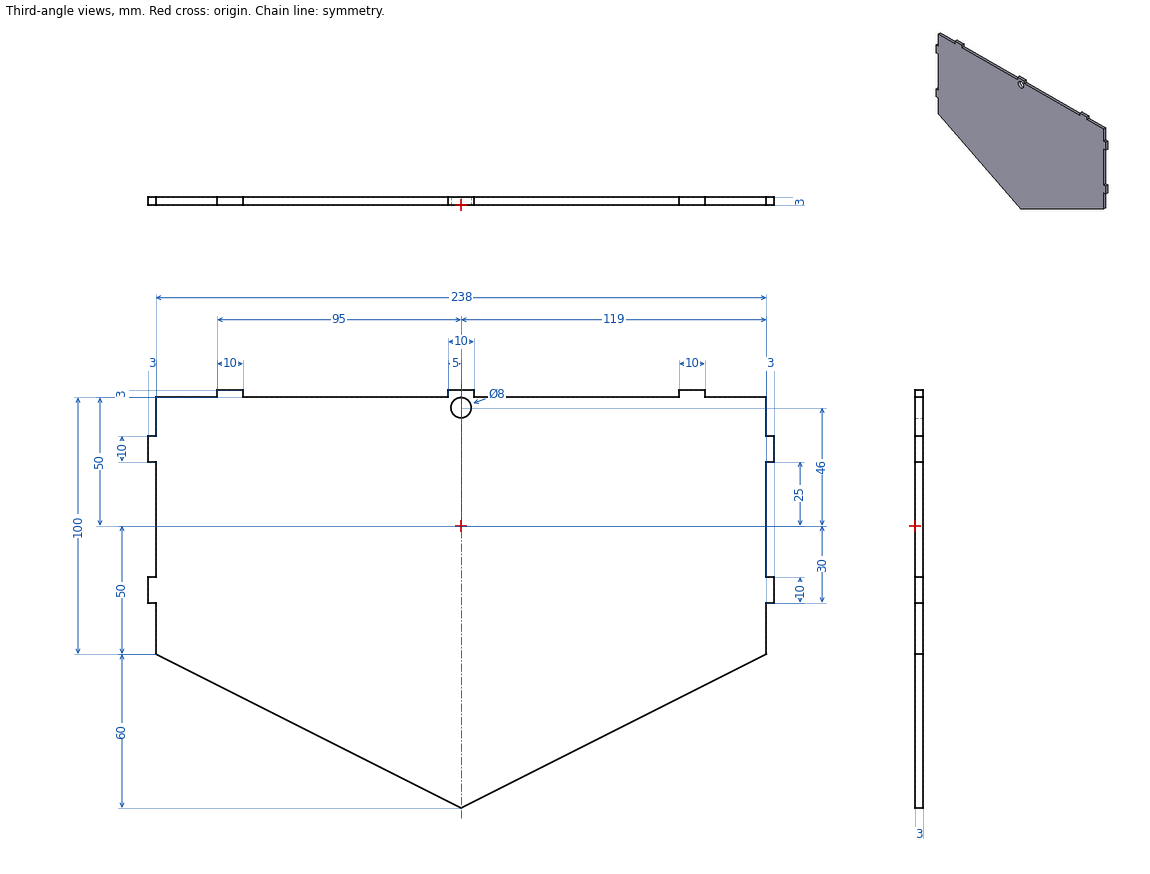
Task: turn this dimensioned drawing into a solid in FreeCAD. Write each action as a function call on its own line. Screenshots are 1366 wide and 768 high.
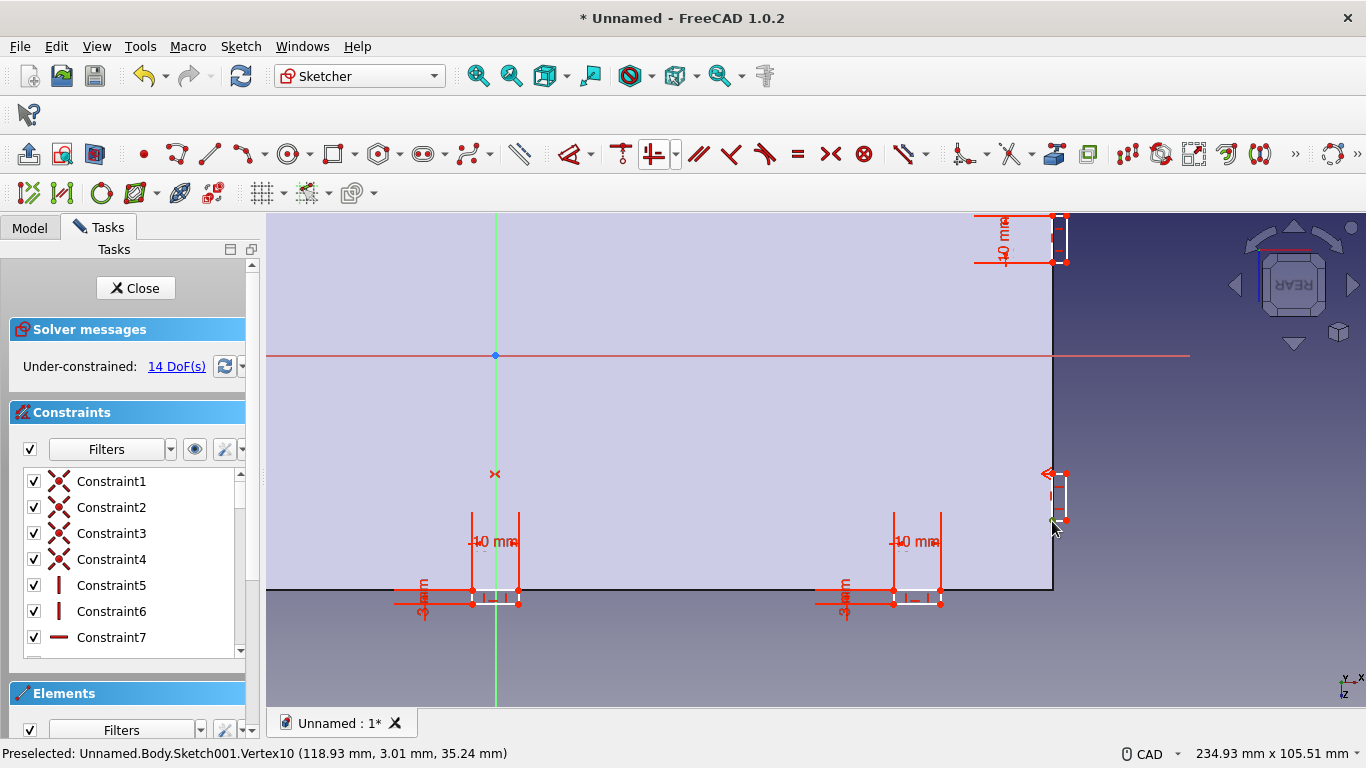
scroll(1054, 521, down, 3)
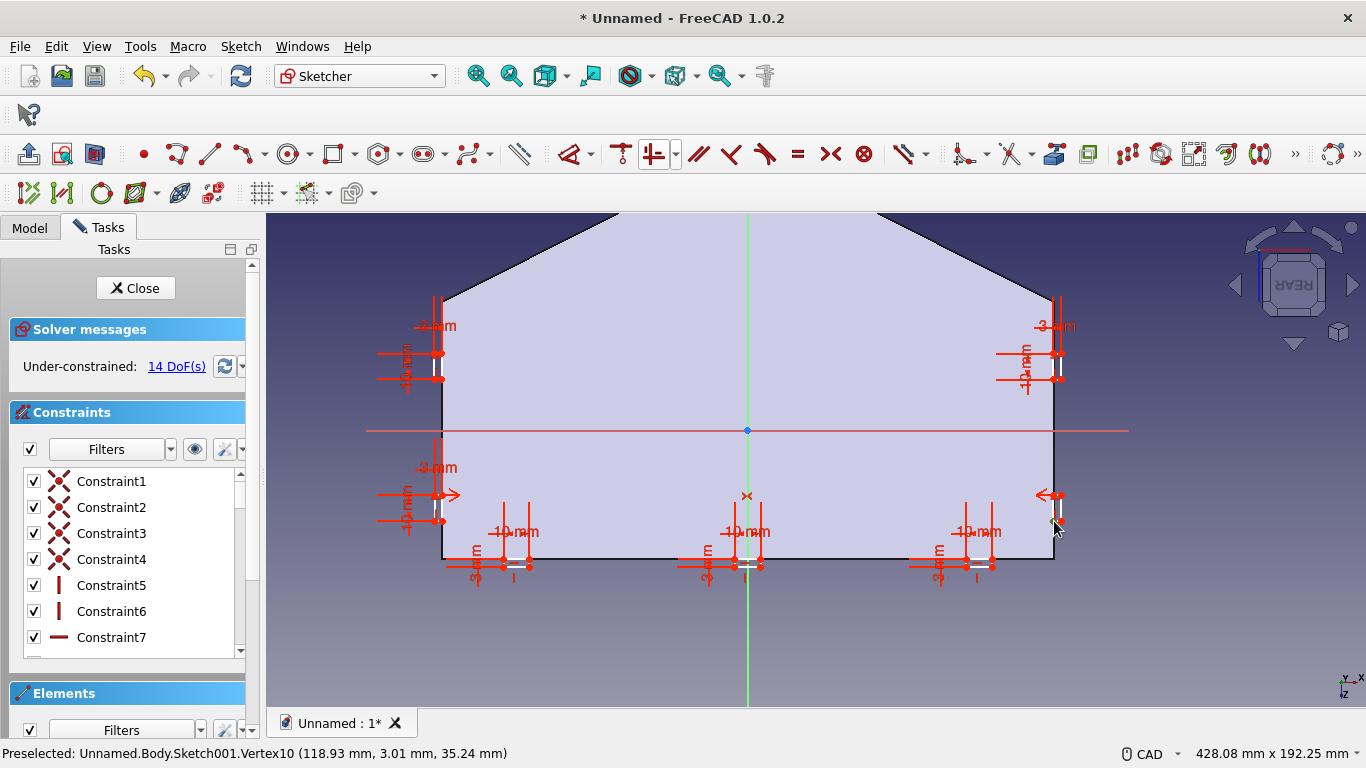
scroll(442, 521, up, 3)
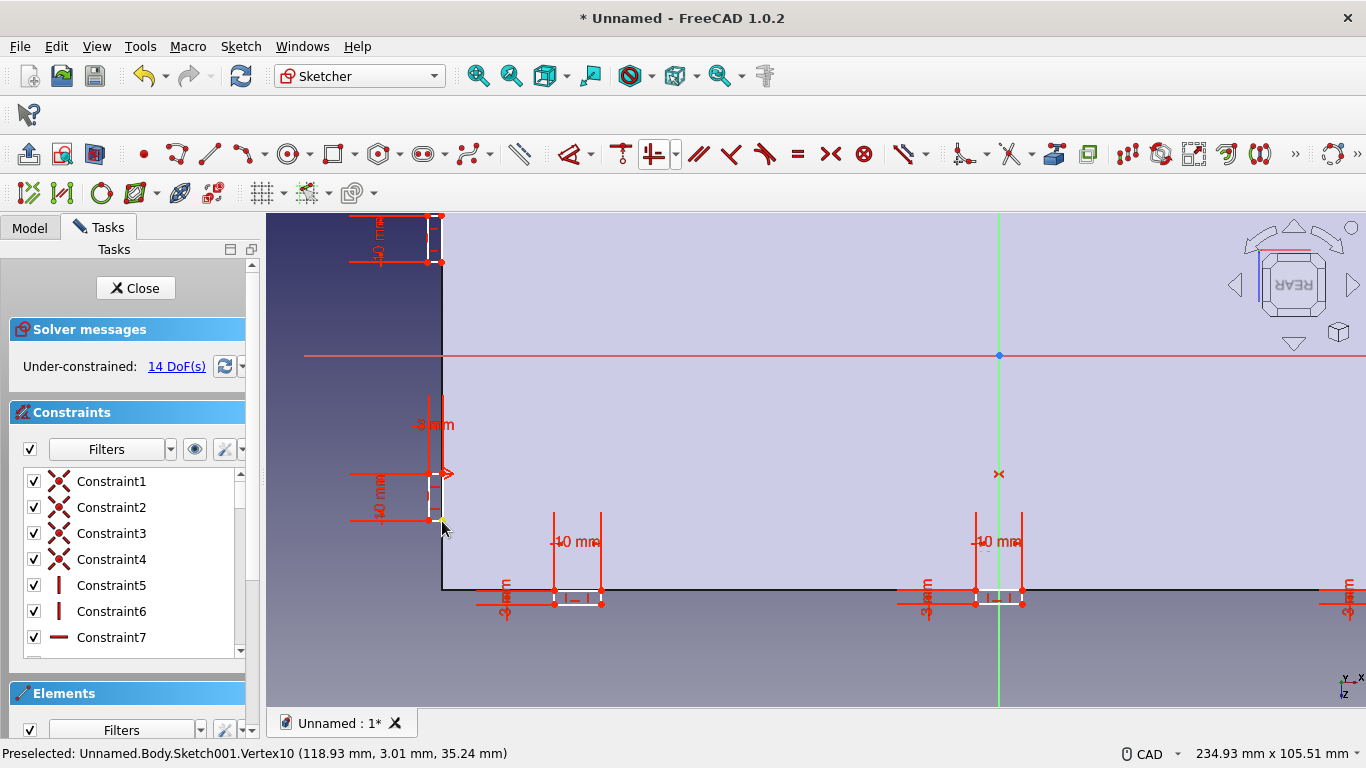
click(443, 521)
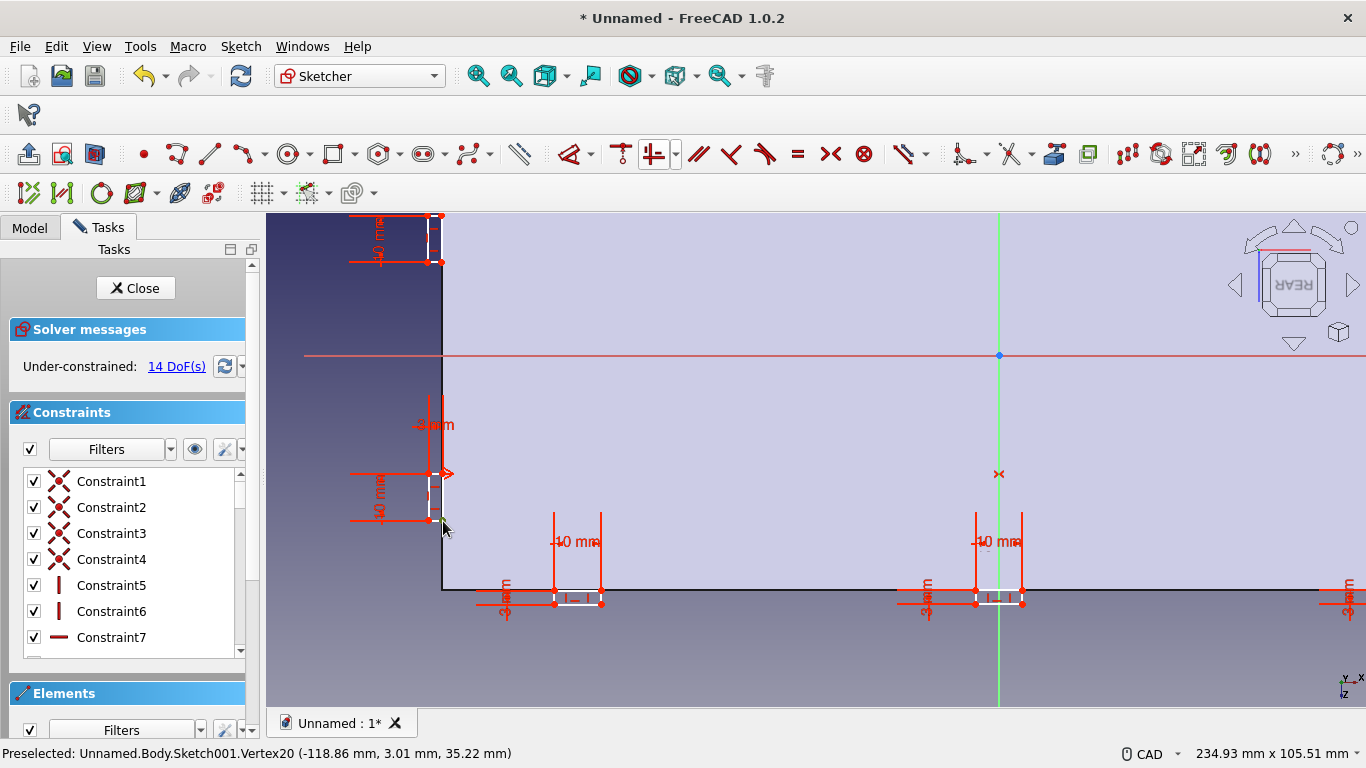
click(999, 648)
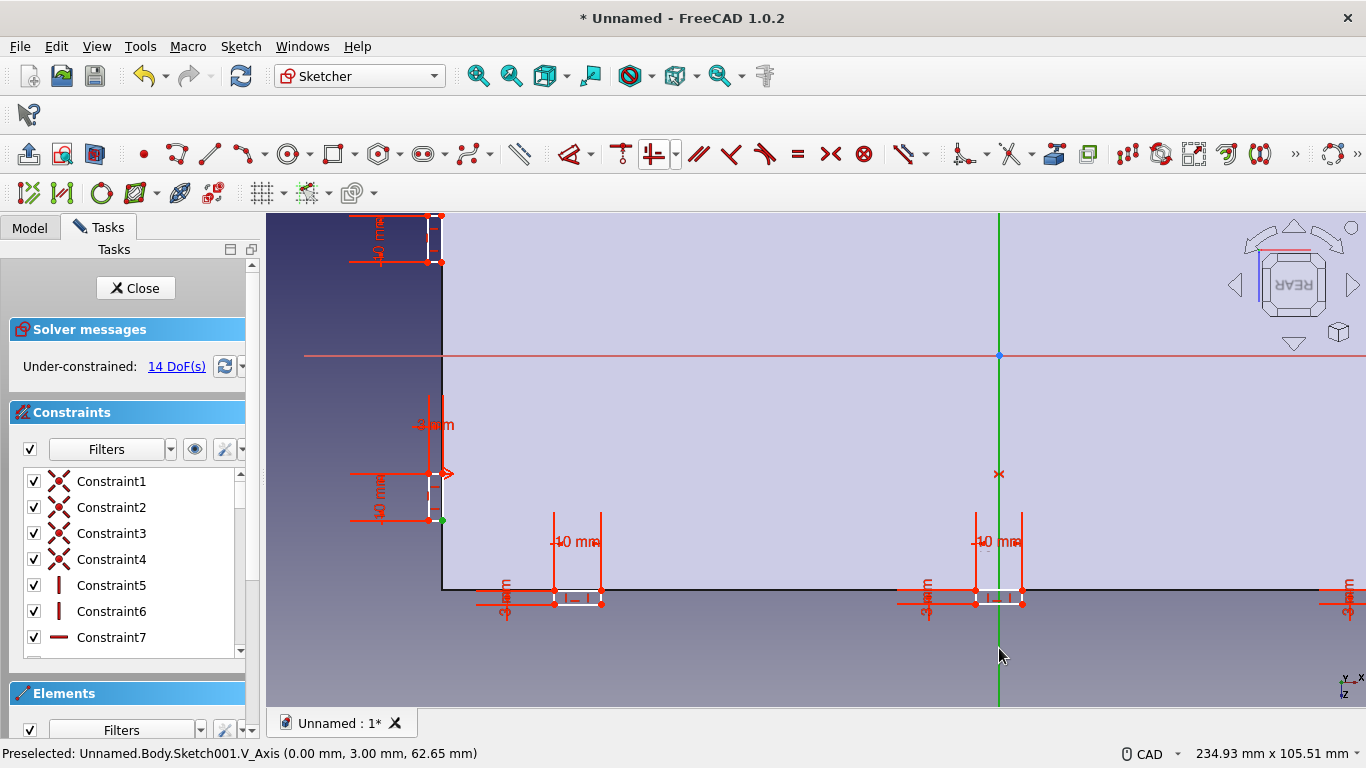
click(831, 154)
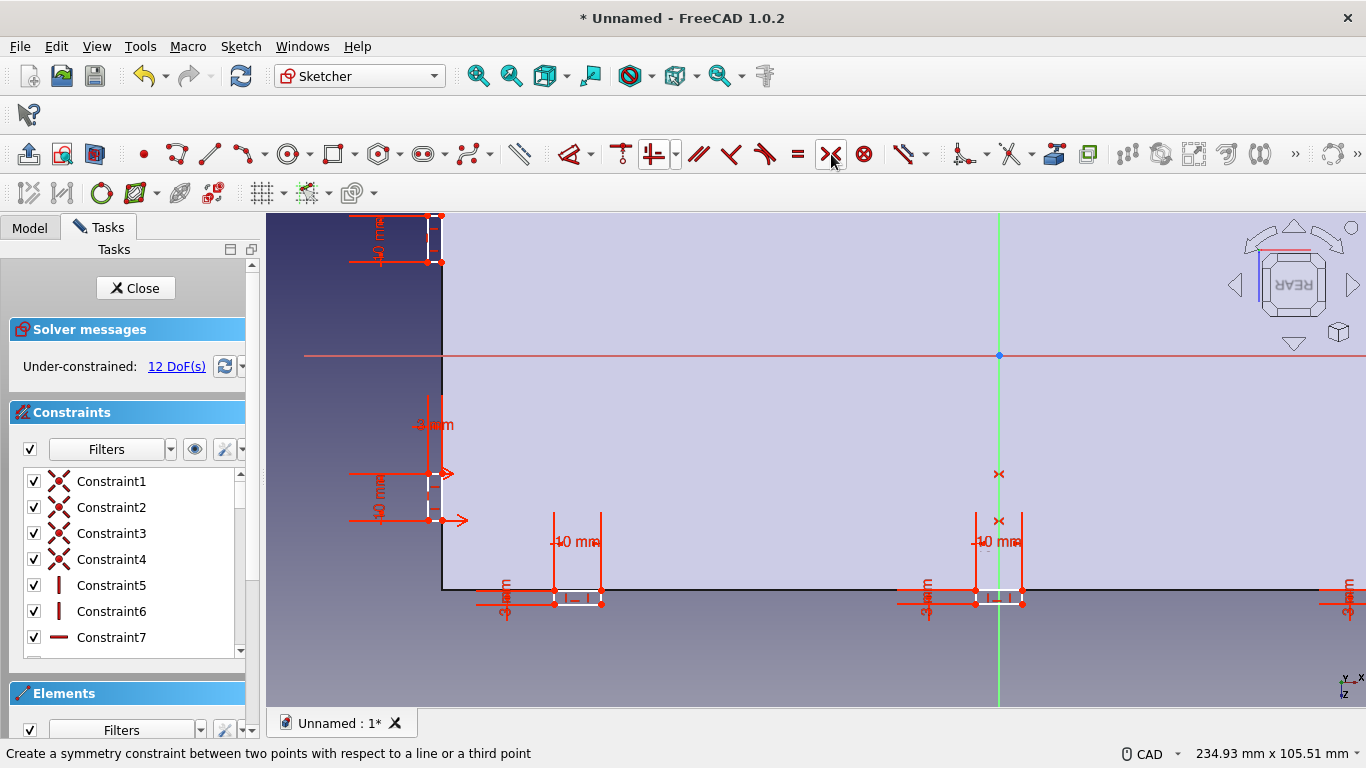
scroll(441, 521, down, 3)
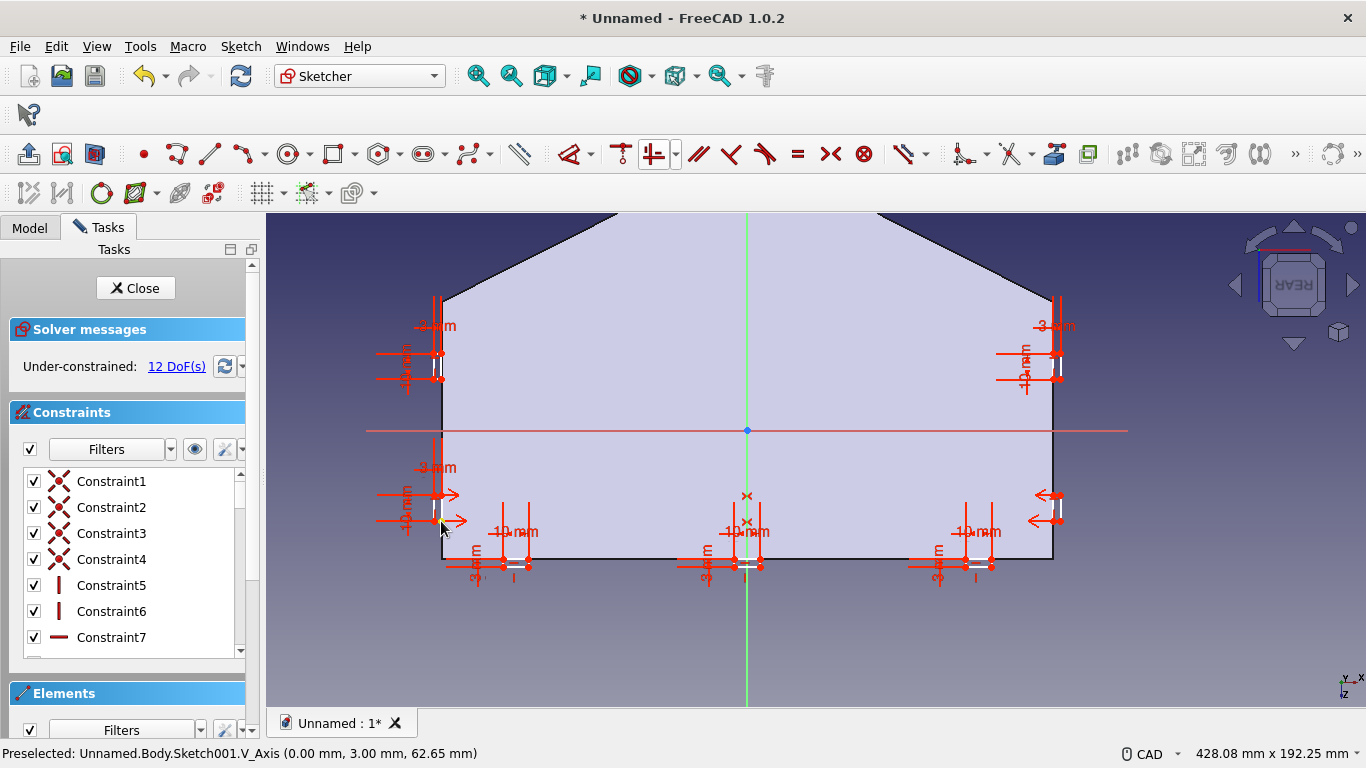
scroll(1061, 354, up, 3)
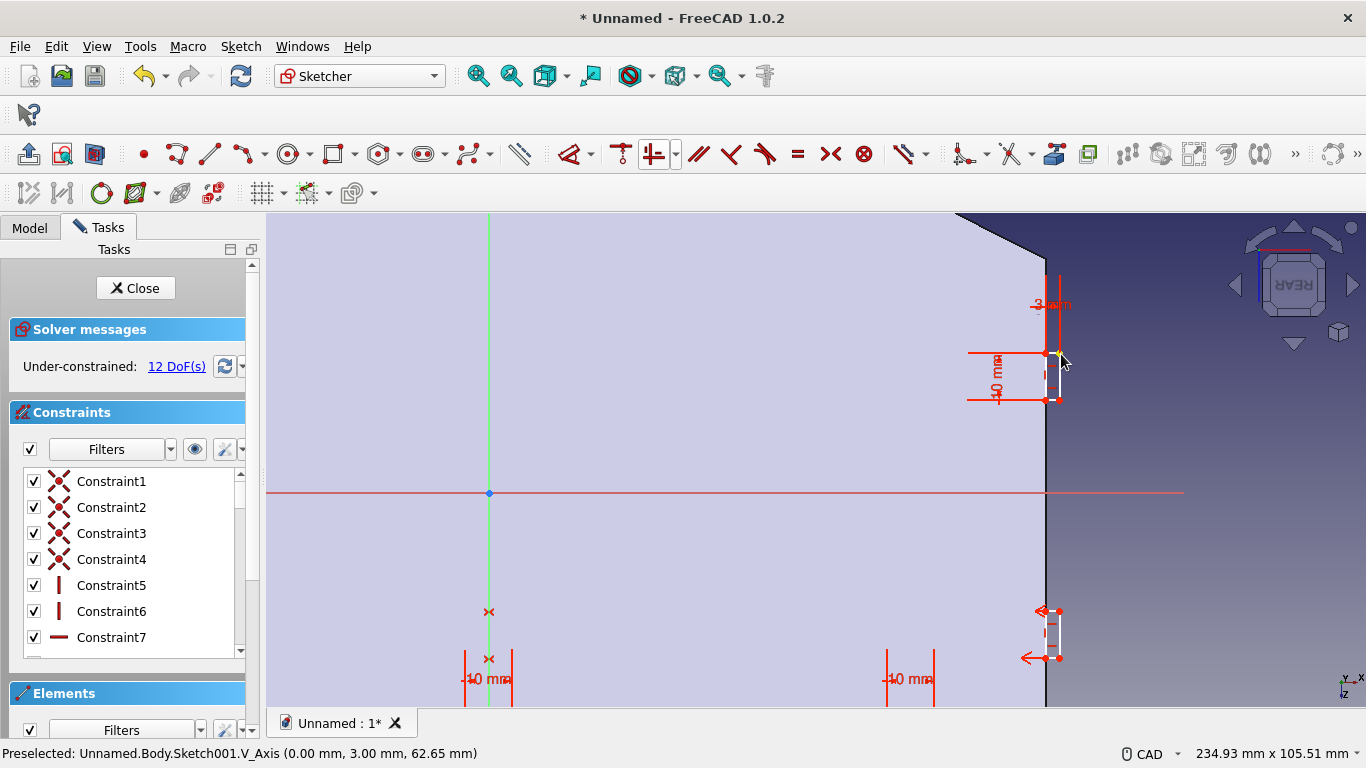
click(1060, 353)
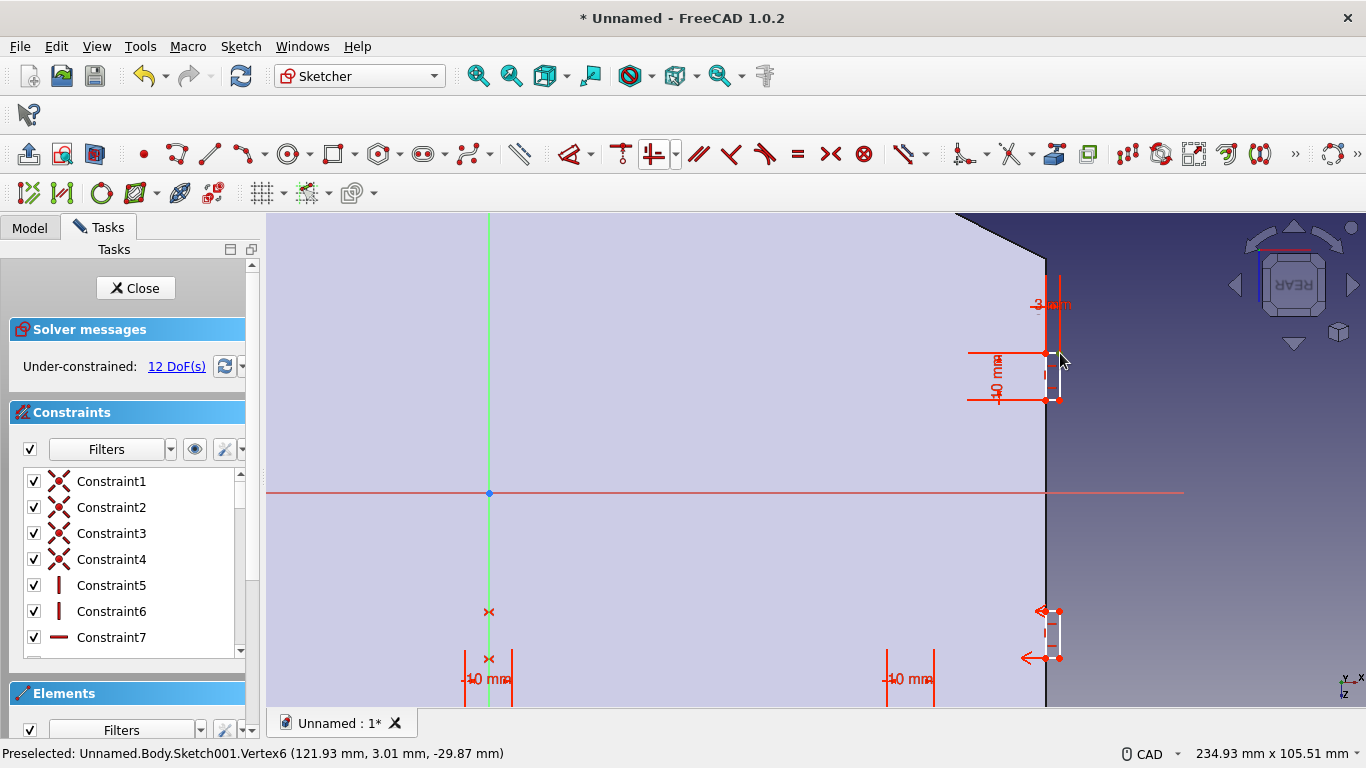
scroll(1062, 354, down, 3)